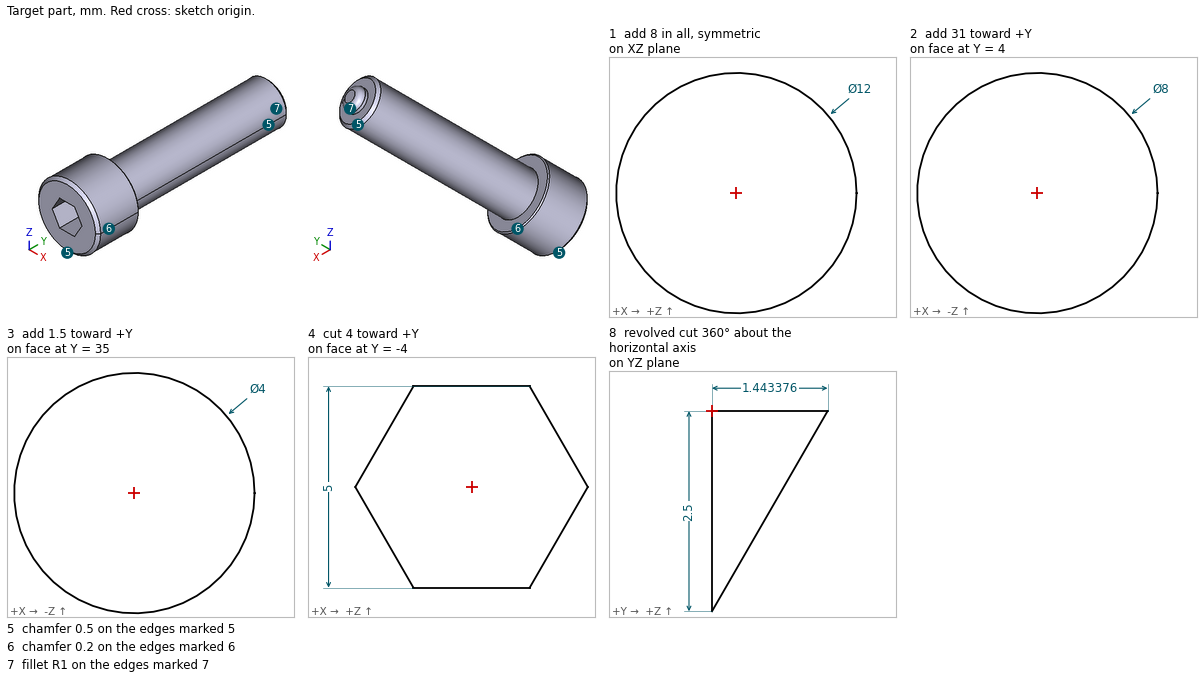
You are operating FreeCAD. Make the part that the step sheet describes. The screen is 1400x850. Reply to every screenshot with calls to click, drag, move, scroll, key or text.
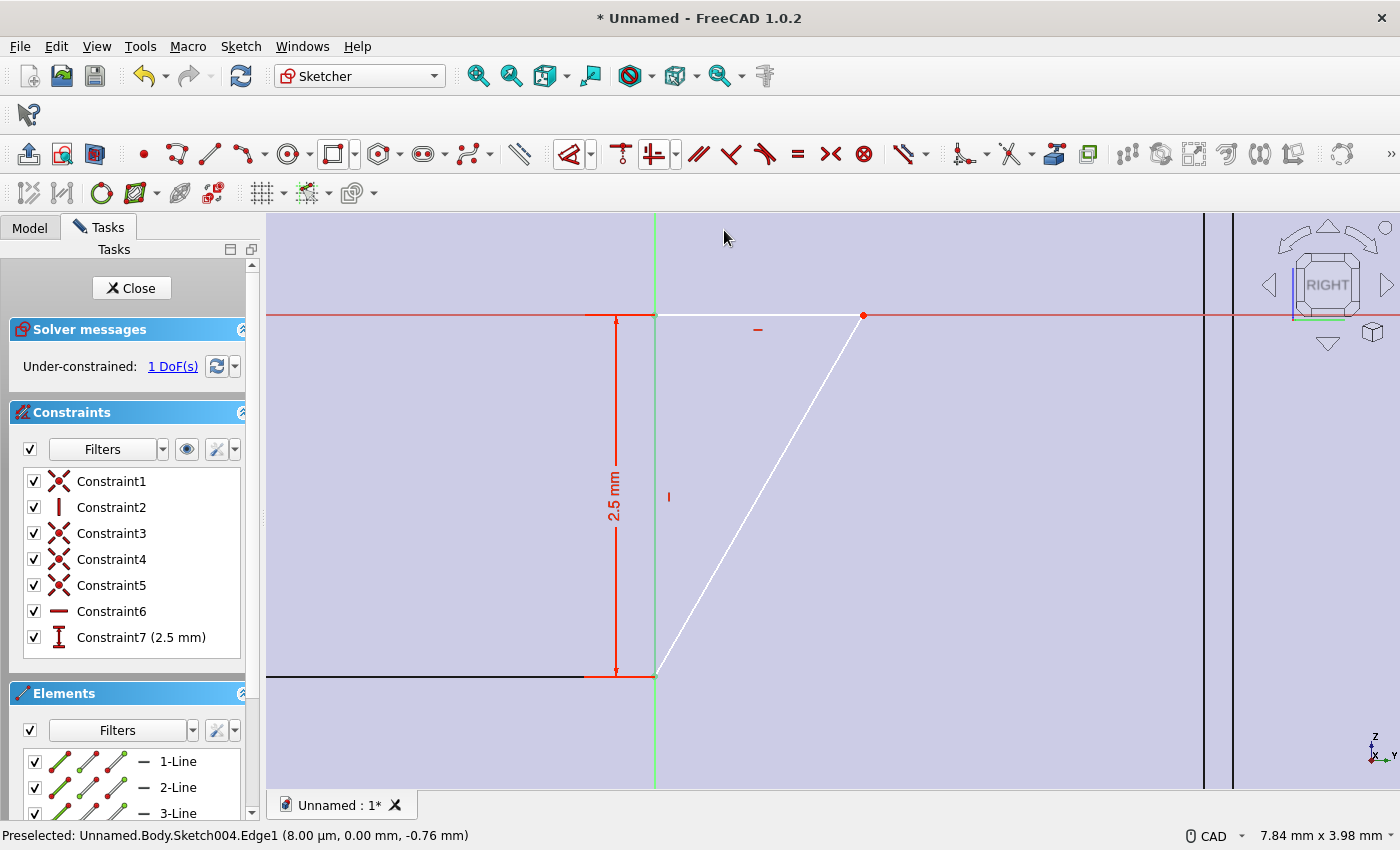
click(801, 315)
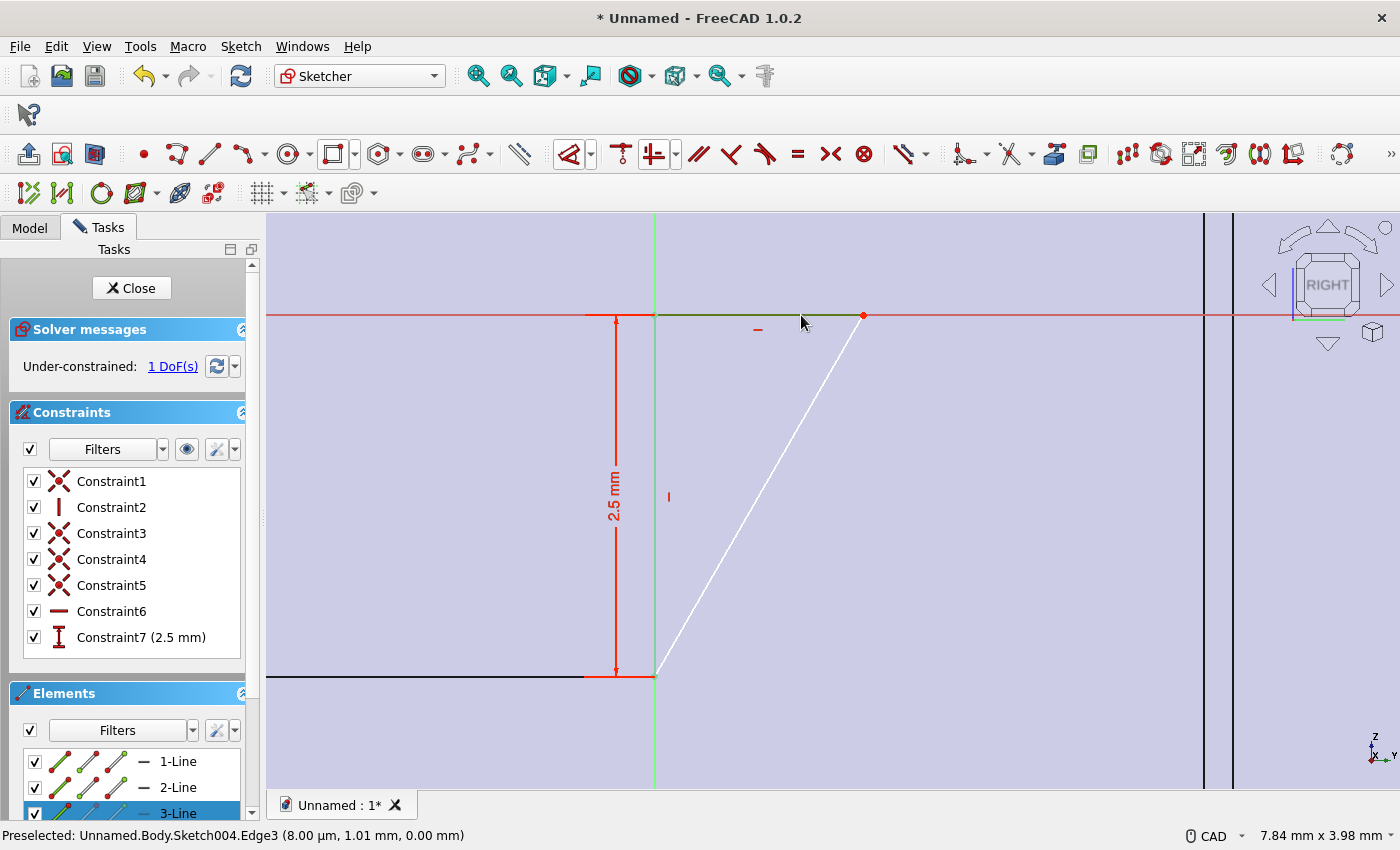
click(590, 154)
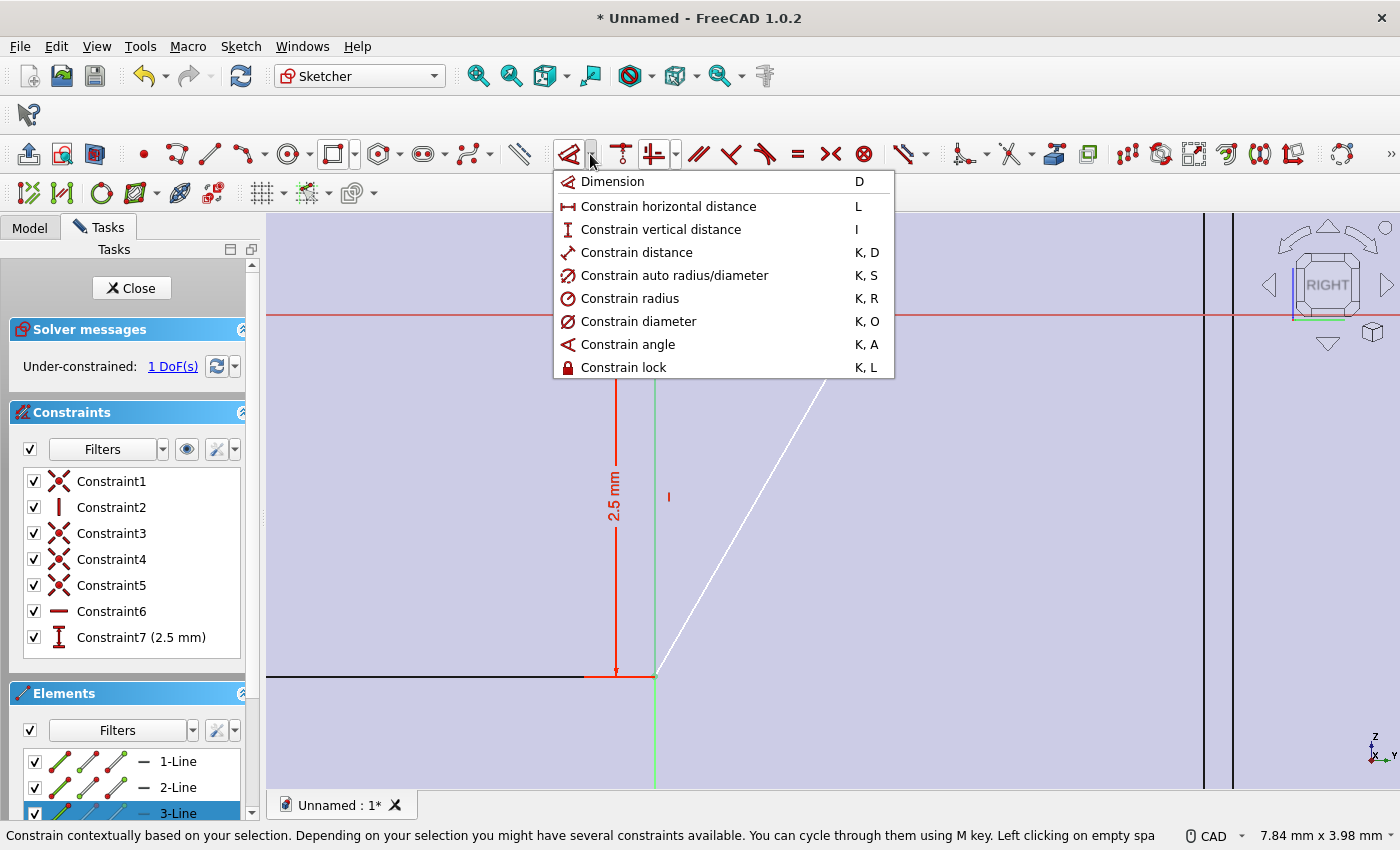
click(724, 206)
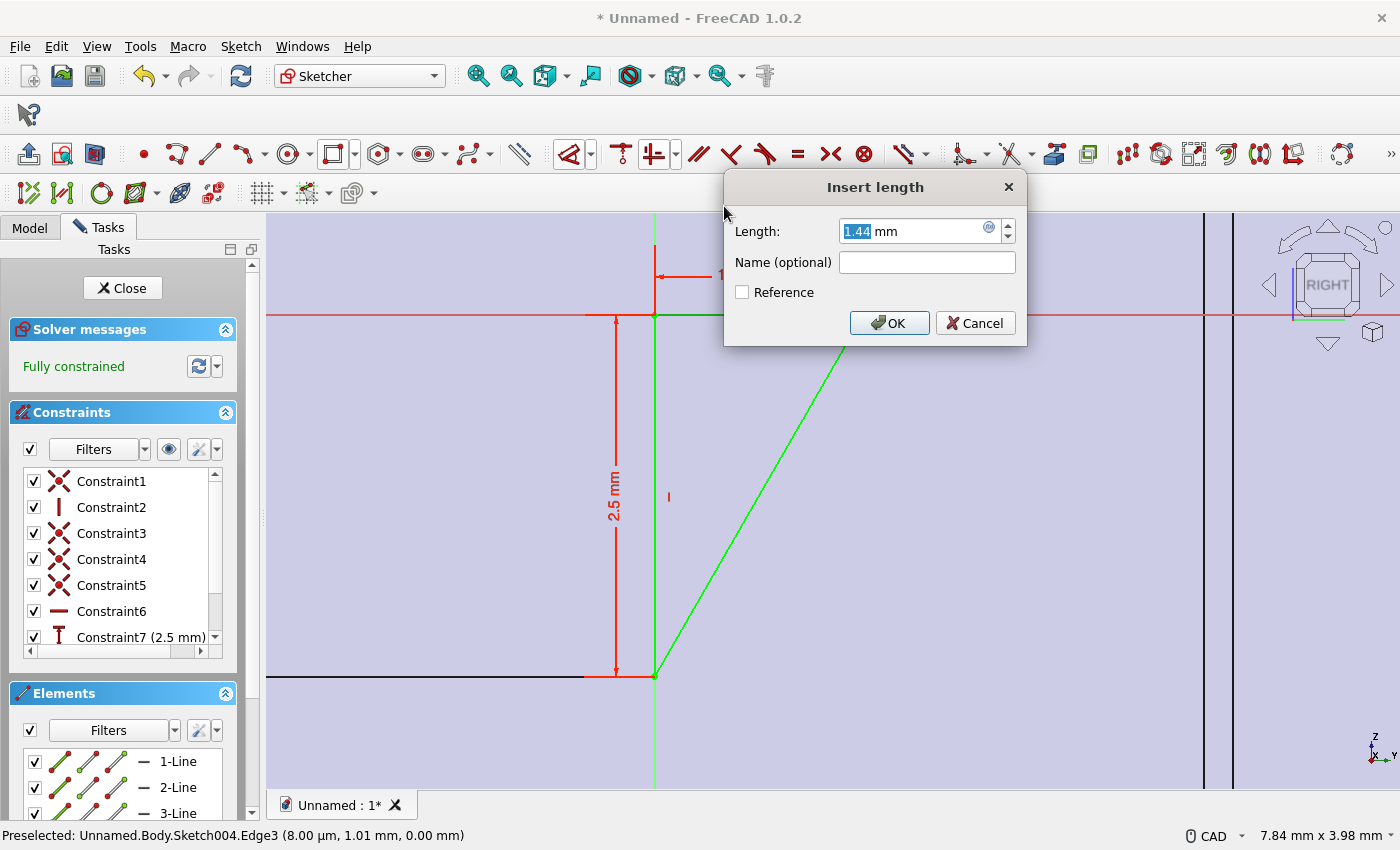
text(1.443376)
key(Return)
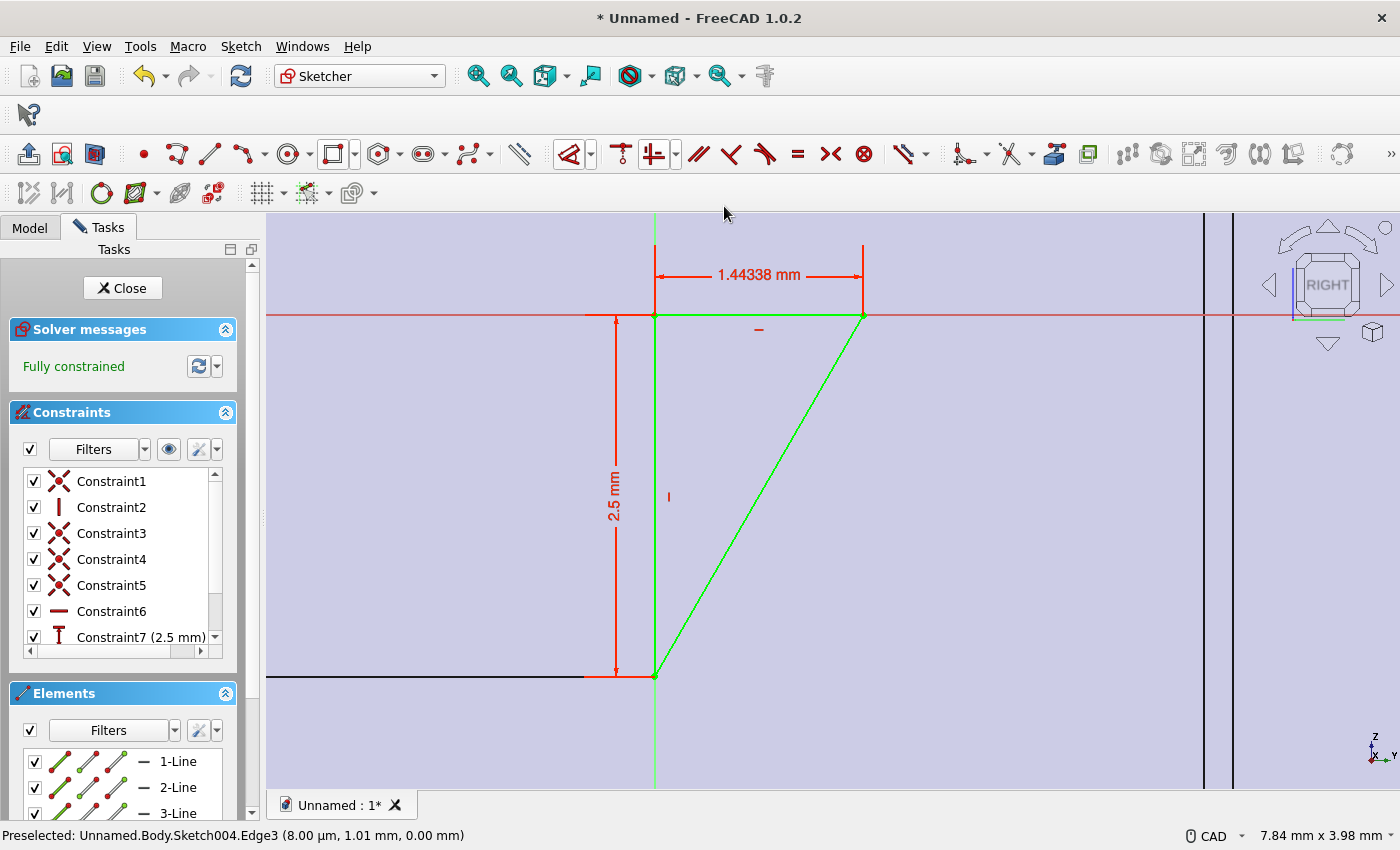
click(123, 288)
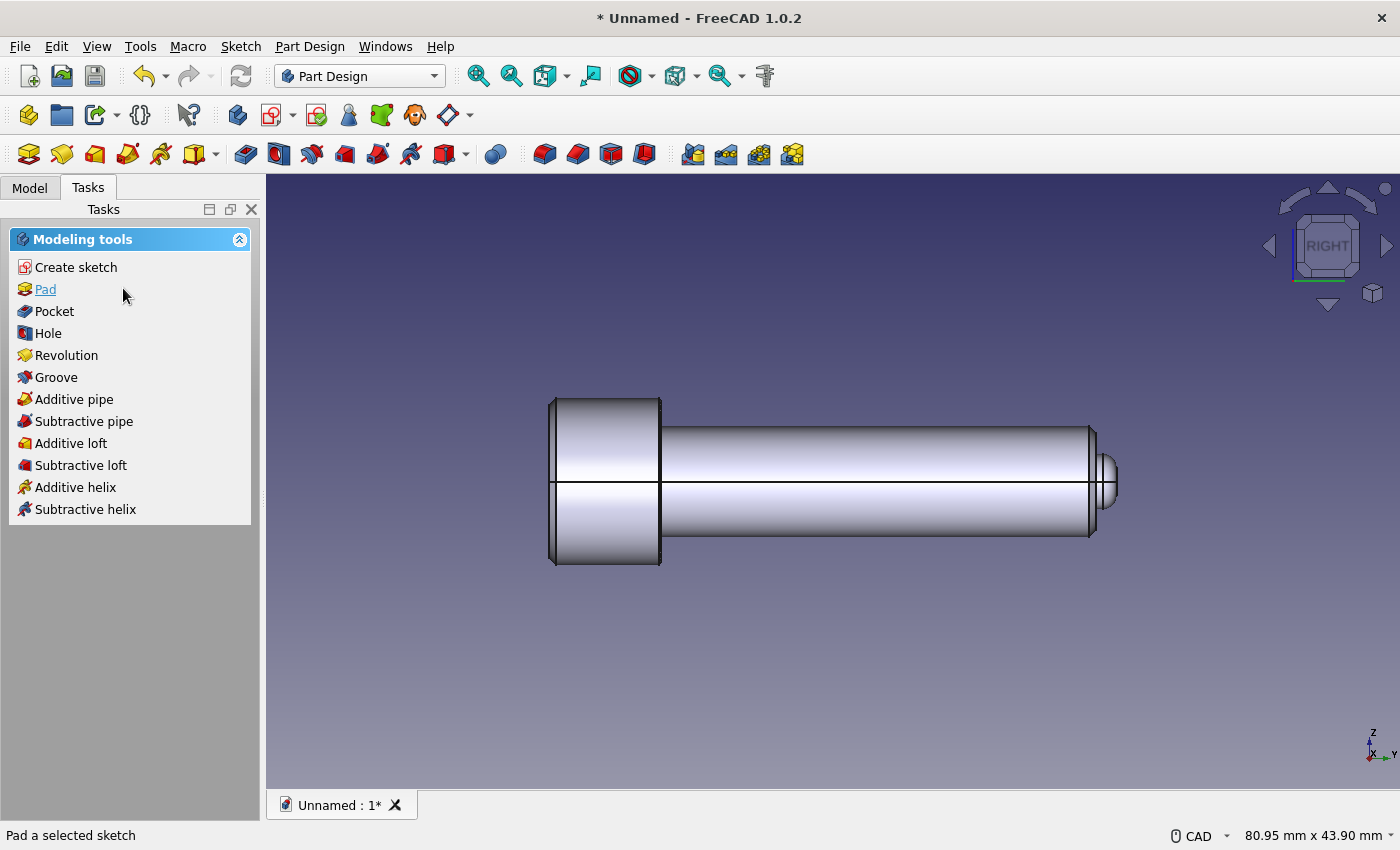
click(312, 154)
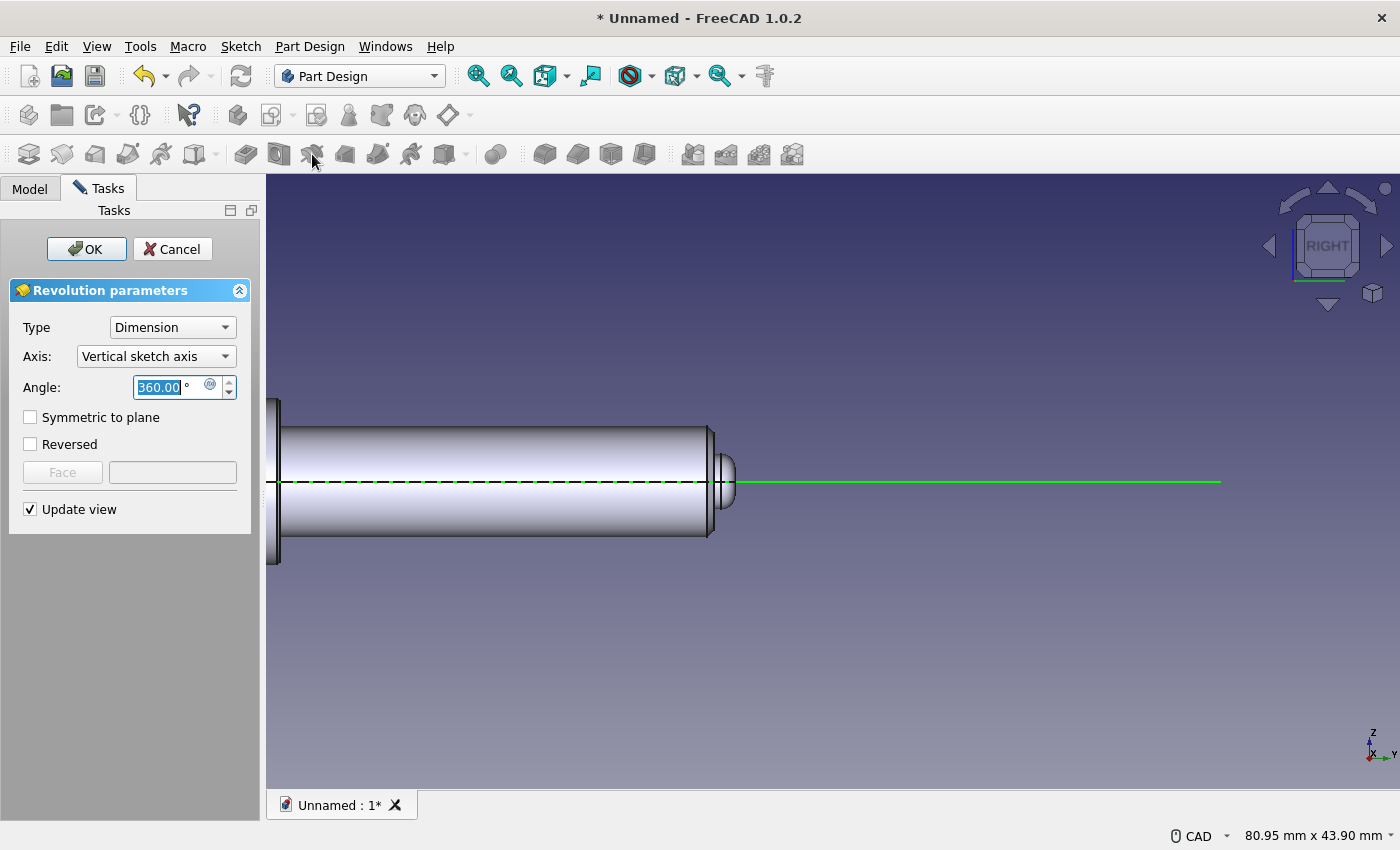
click(157, 356)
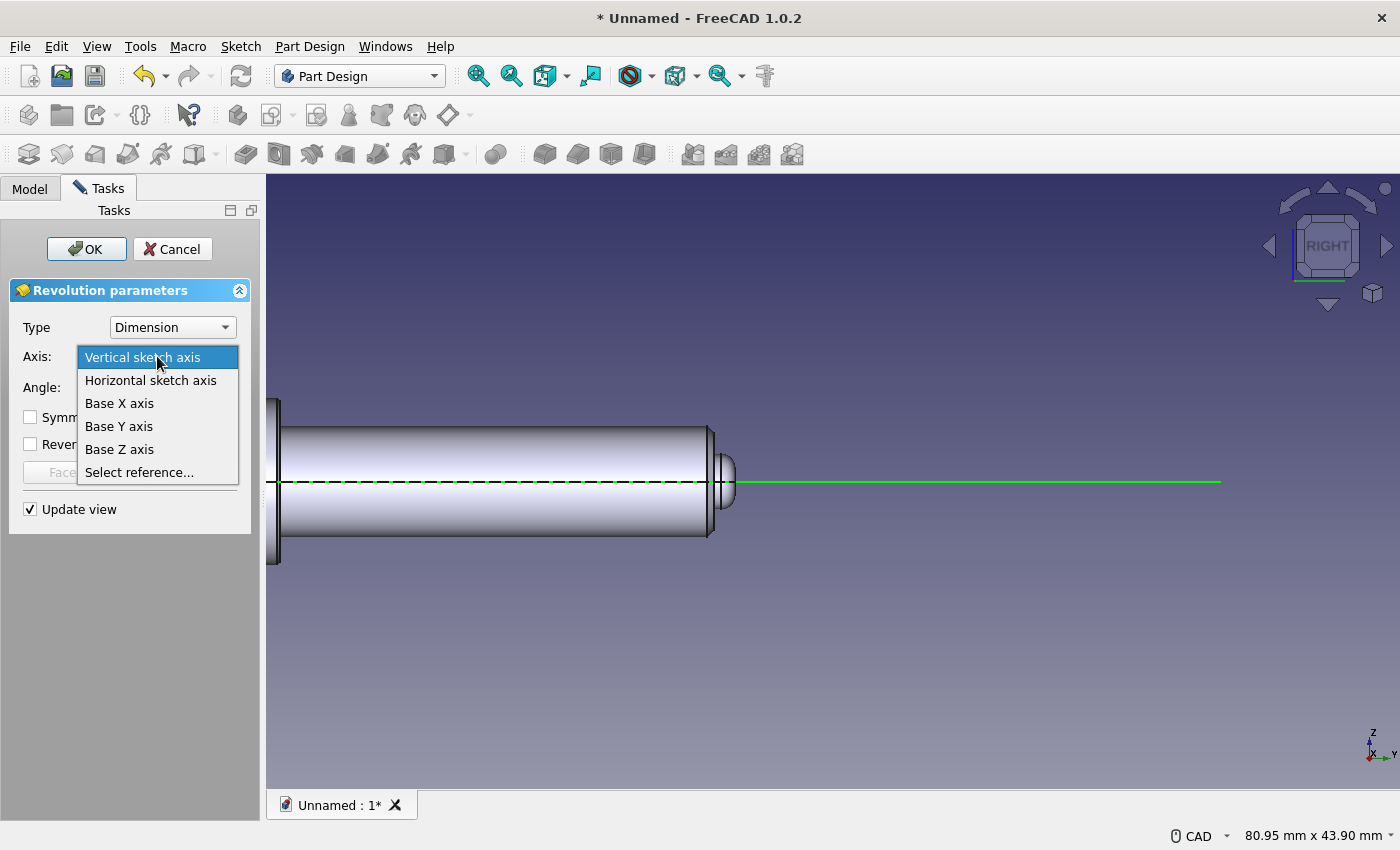
click(156, 380)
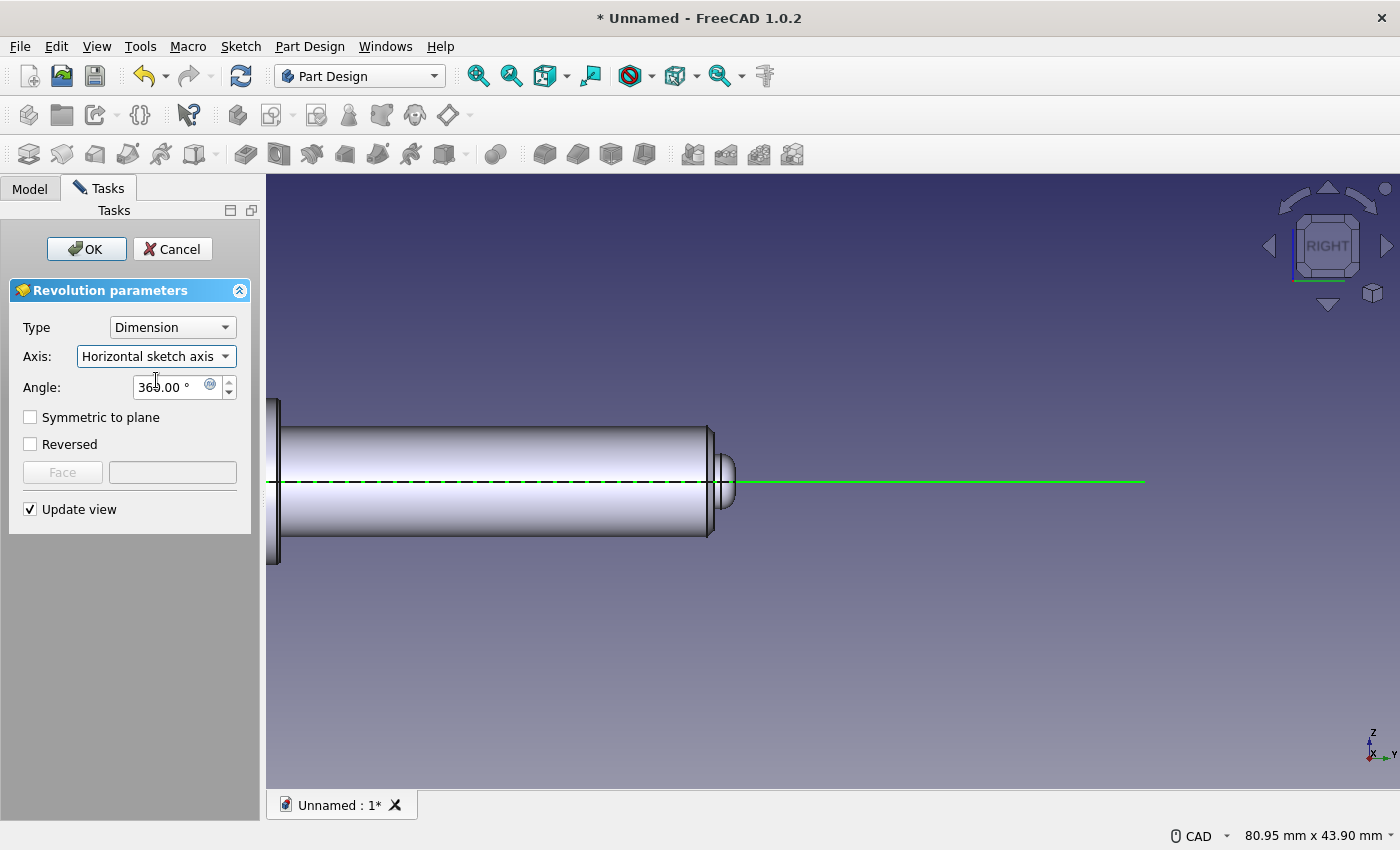
click(87, 249)